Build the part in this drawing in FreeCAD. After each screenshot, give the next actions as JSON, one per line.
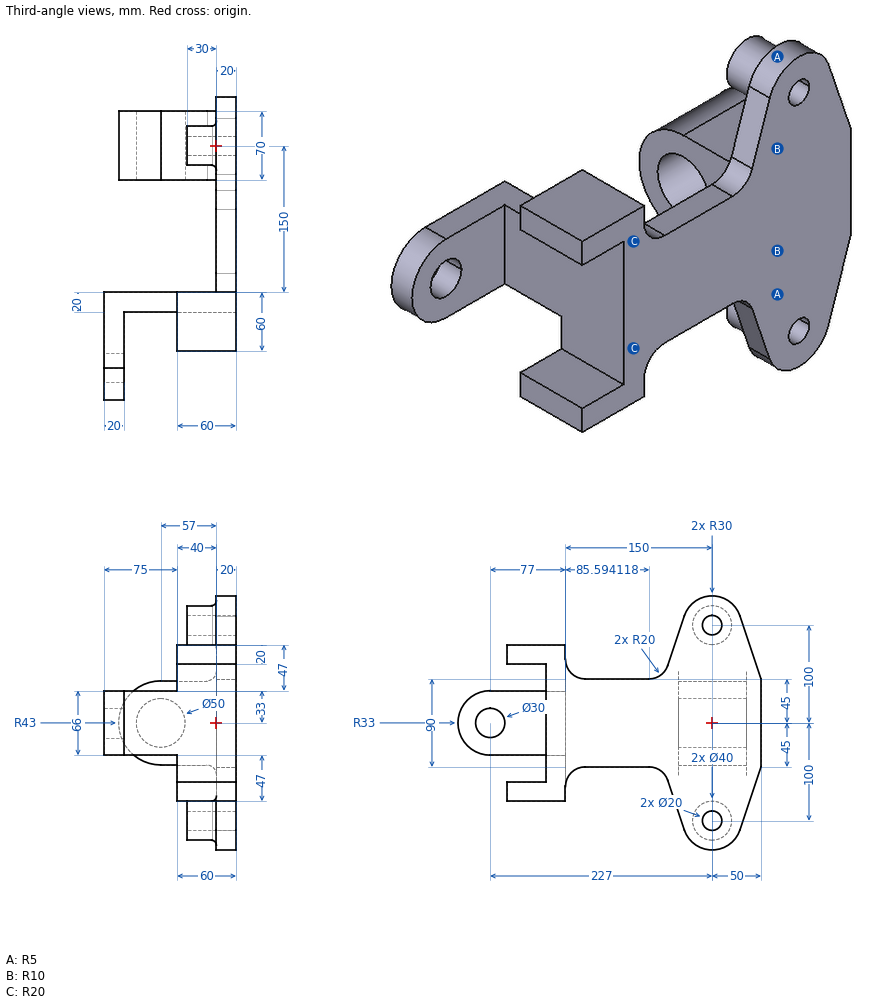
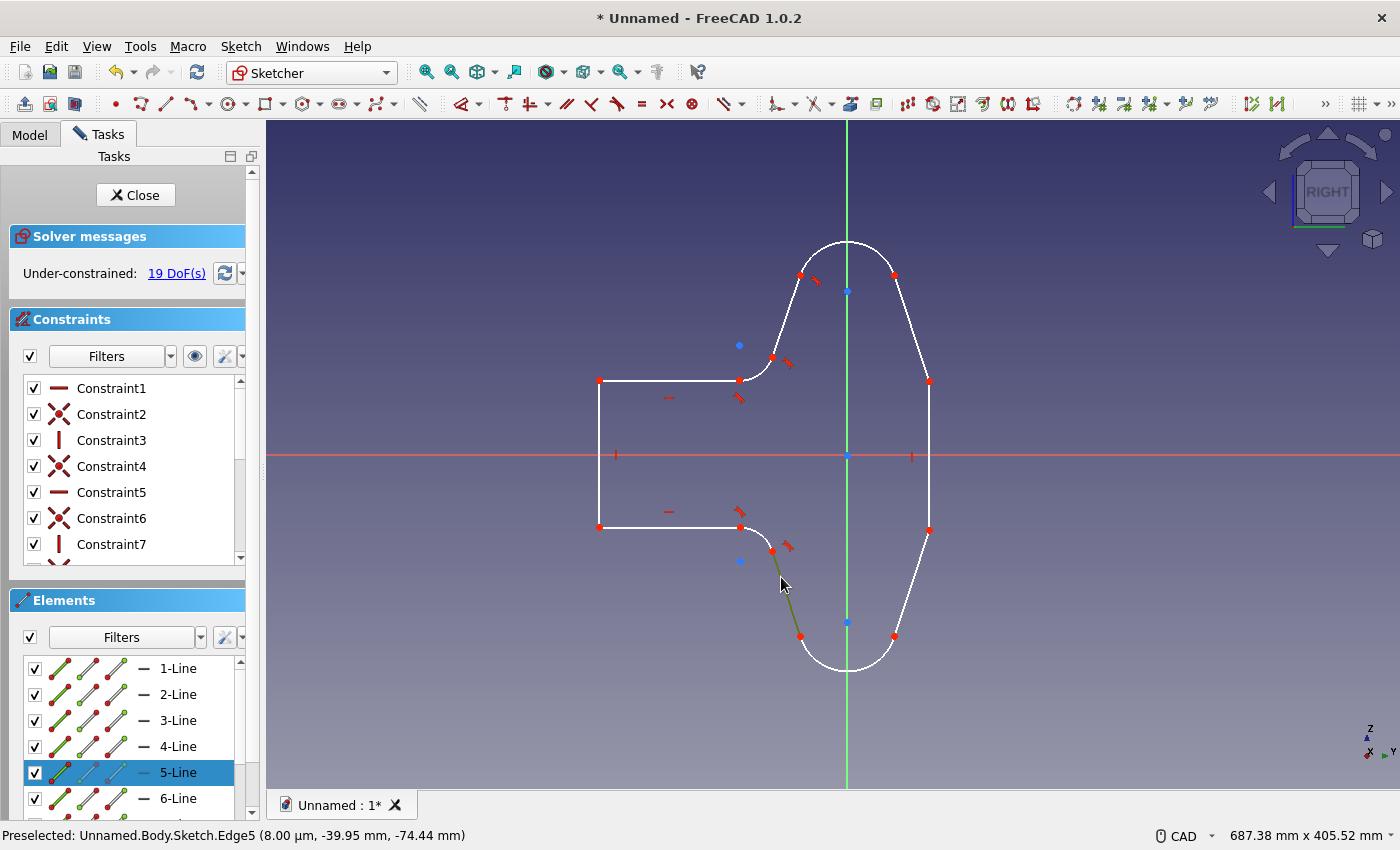
{"action": "left_click", "coordinate": [823, 665]}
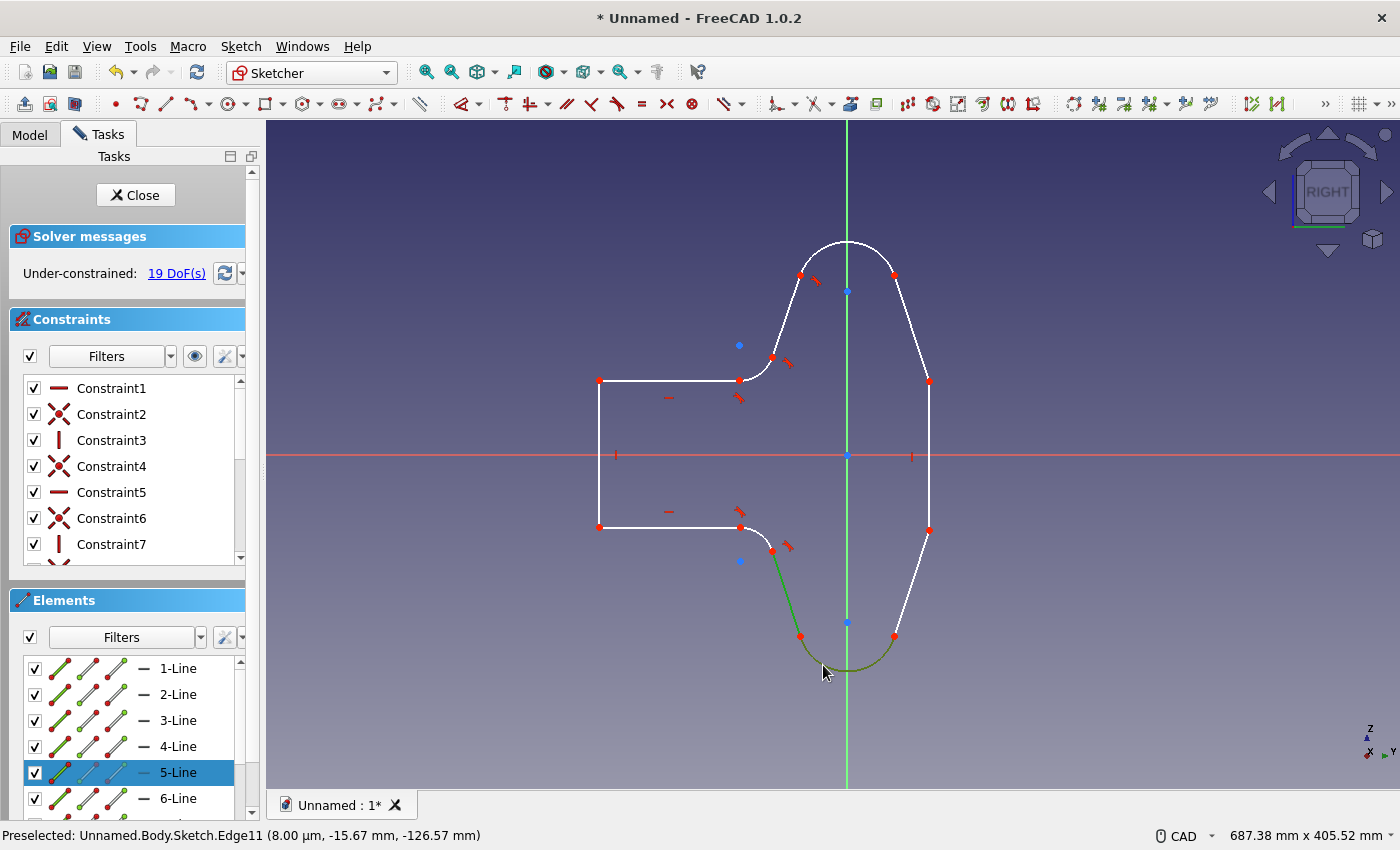
{"action": "left_click", "coordinate": [617, 104]}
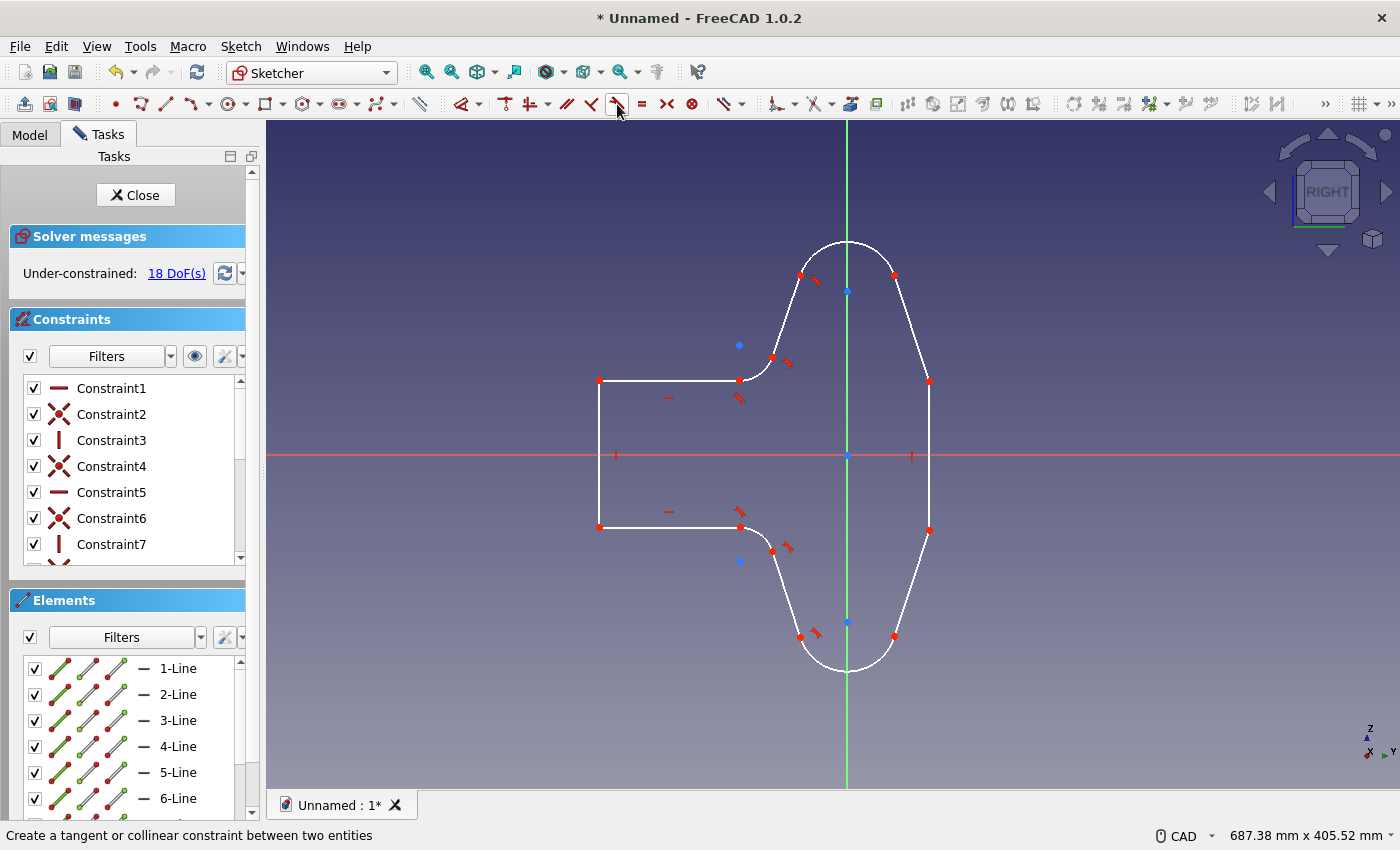
{"action": "left_click", "coordinate": [905, 605]}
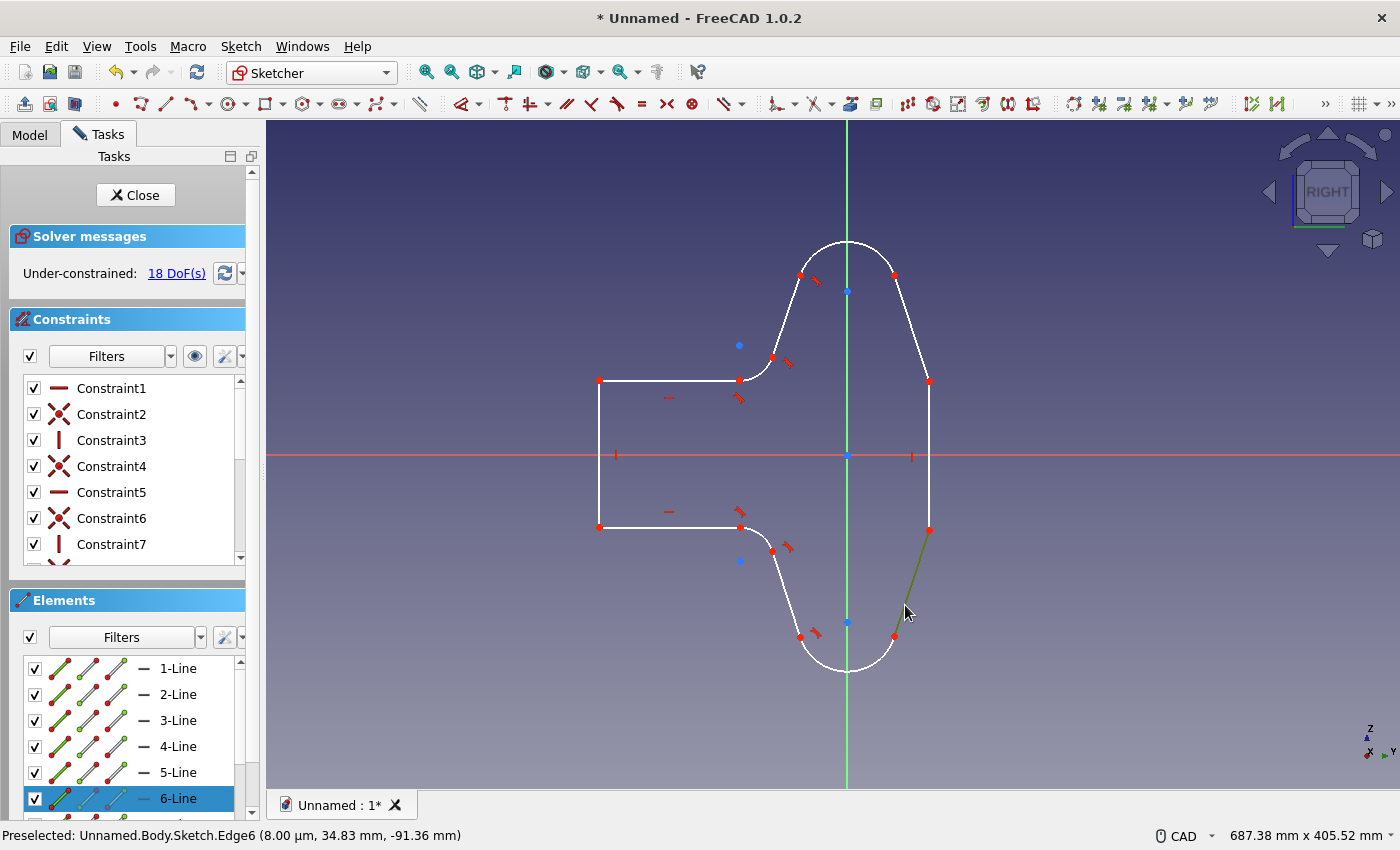
{"action": "left_click", "coordinate": [824, 666]}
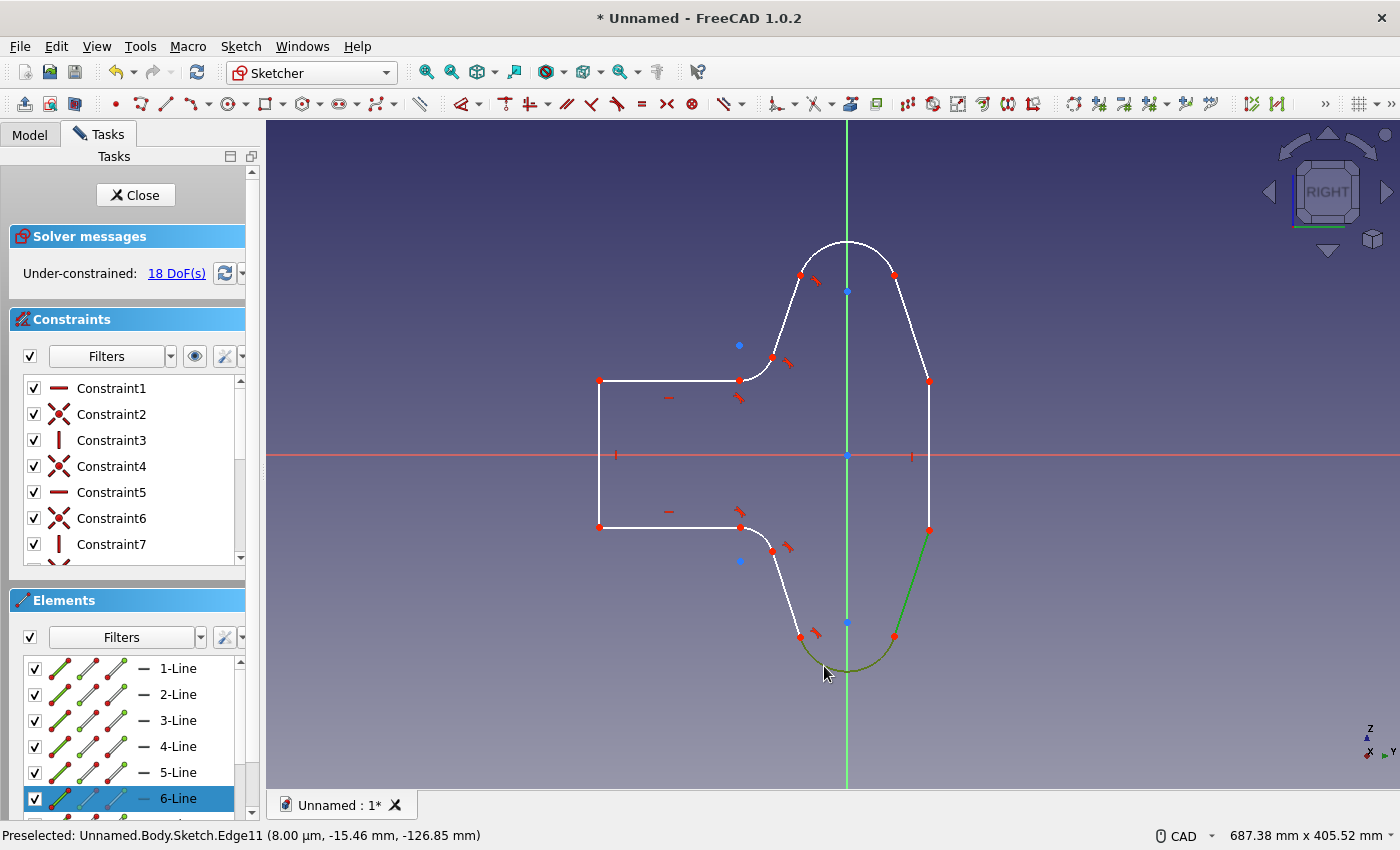
{"action": "left_click", "coordinate": [617, 104]}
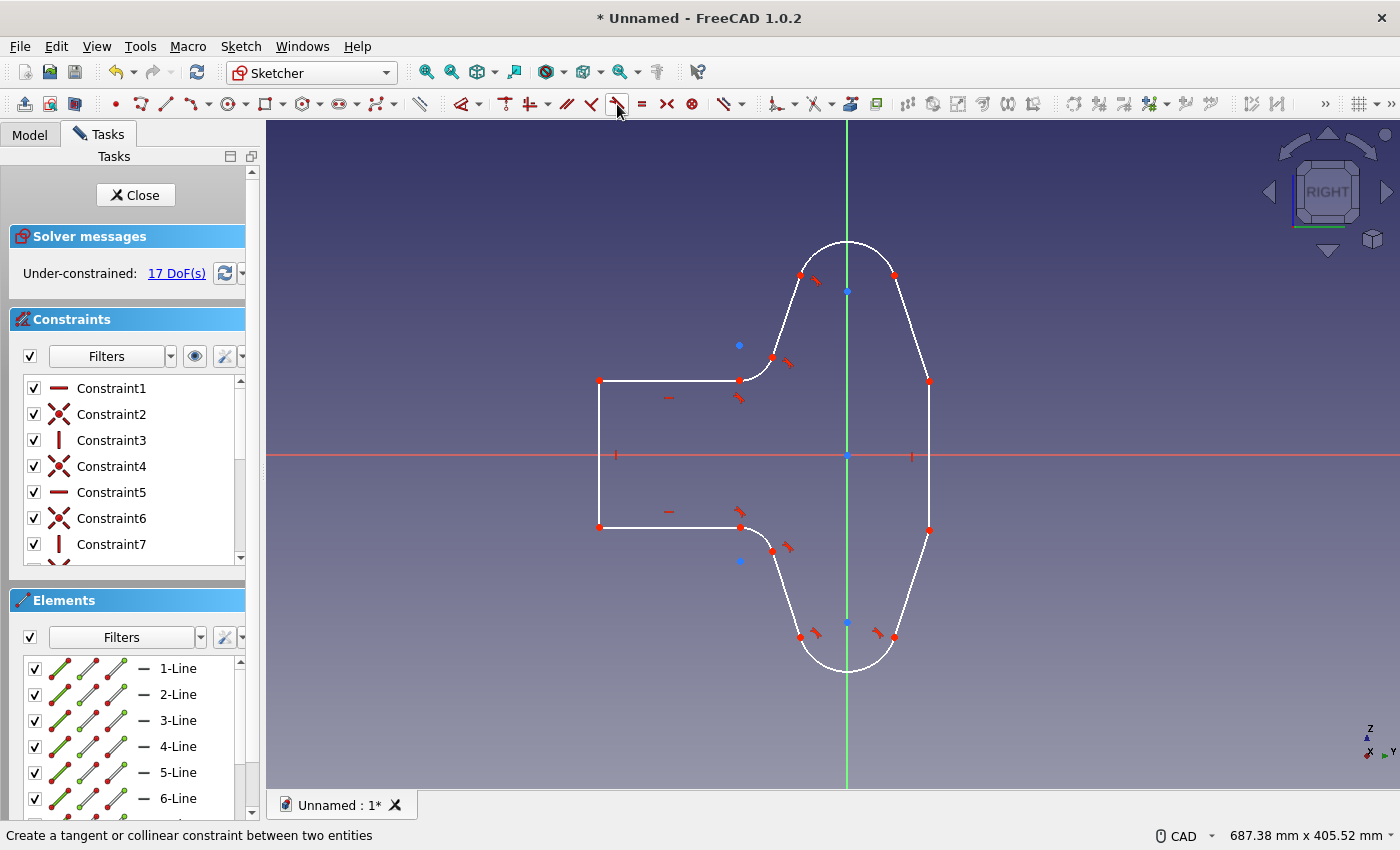
{"action": "left_click", "coordinate": [919, 350]}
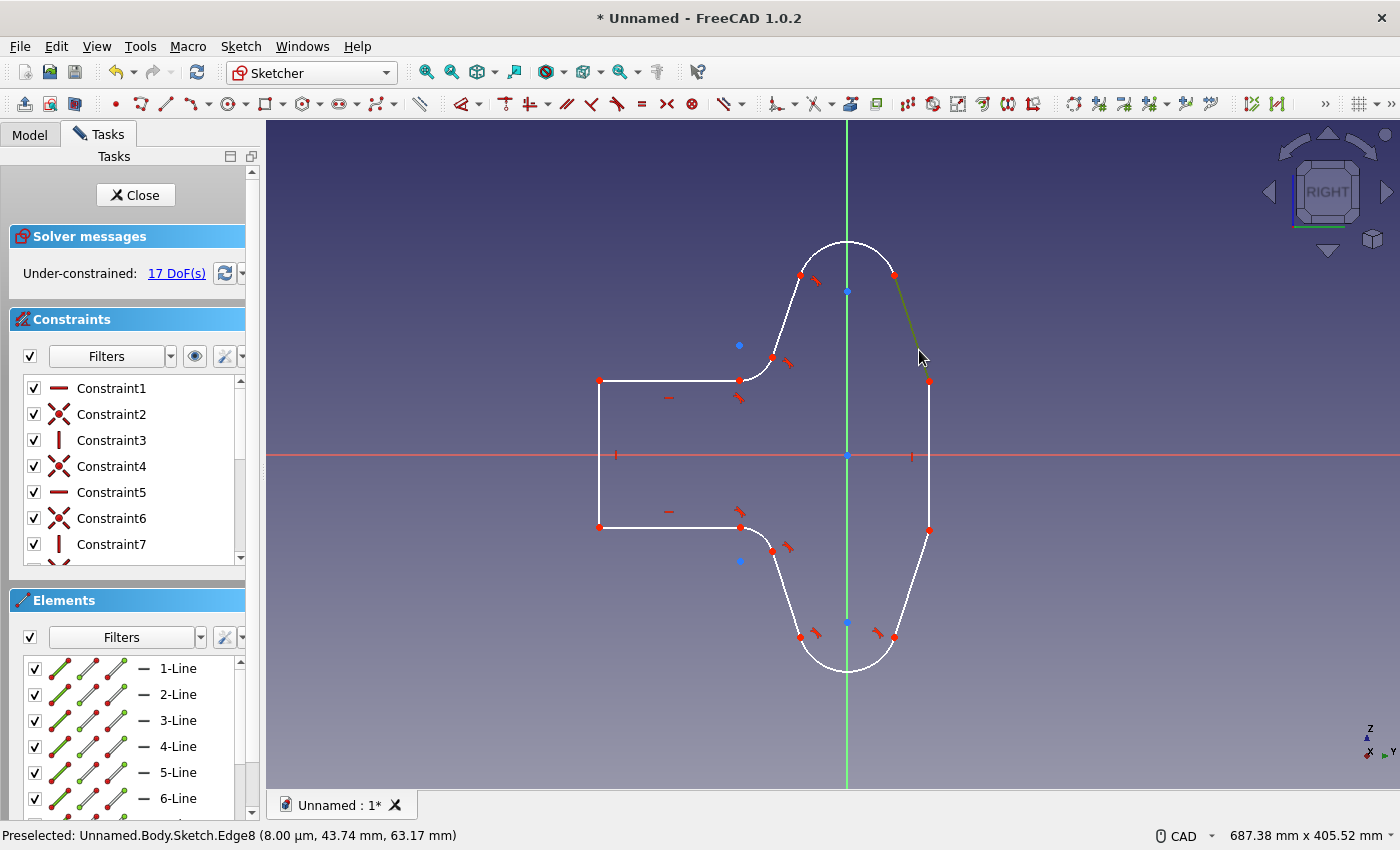
{"action": "left_click", "coordinate": [871, 248]}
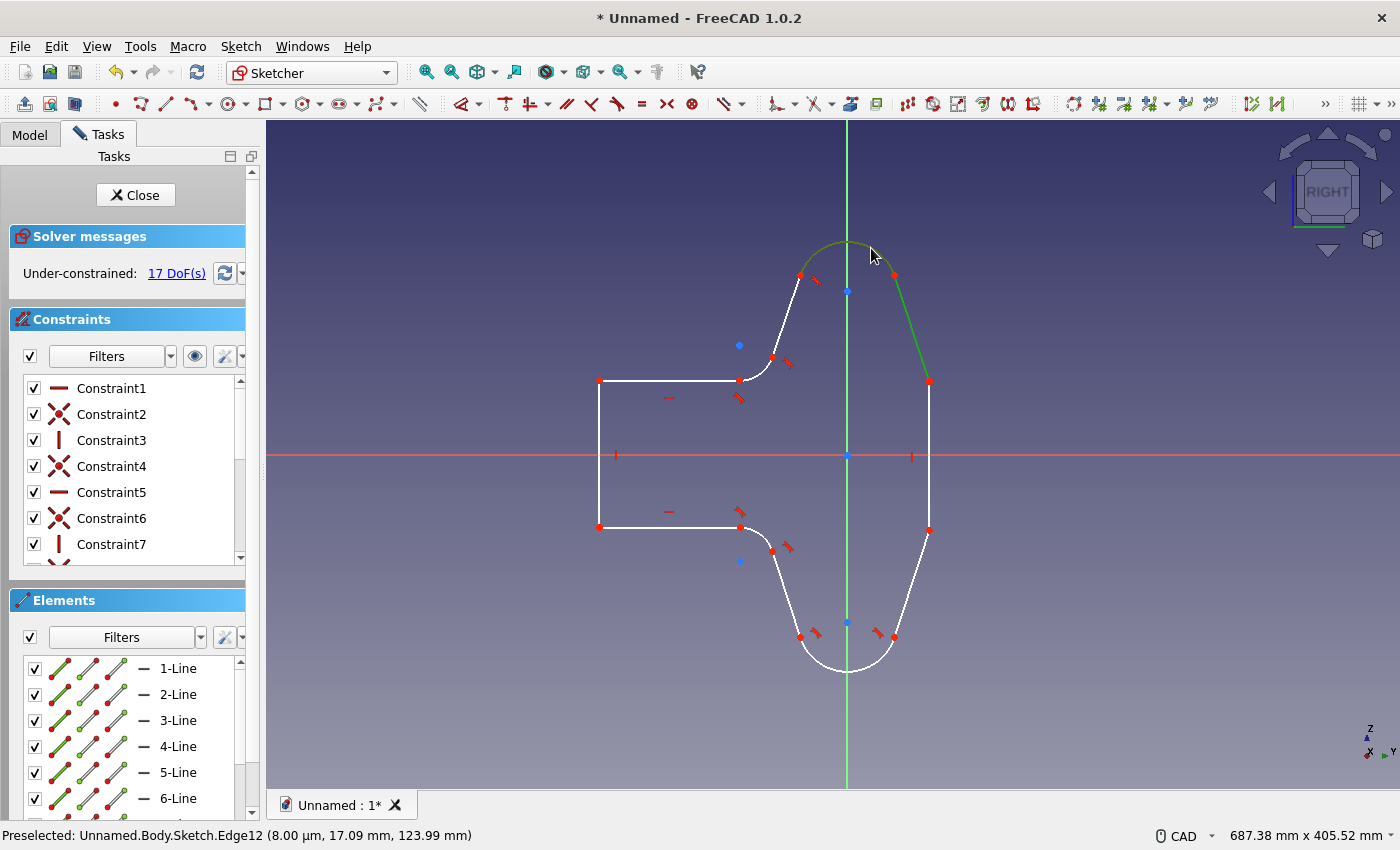
{"action": "key", "text": "t"}